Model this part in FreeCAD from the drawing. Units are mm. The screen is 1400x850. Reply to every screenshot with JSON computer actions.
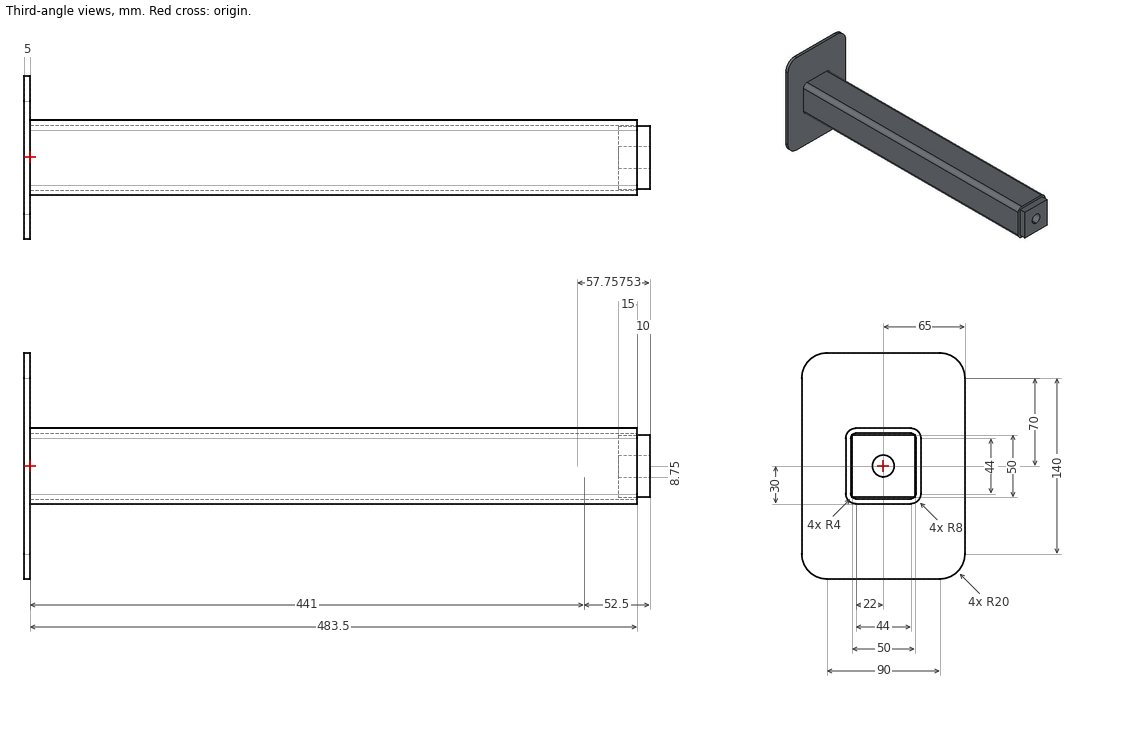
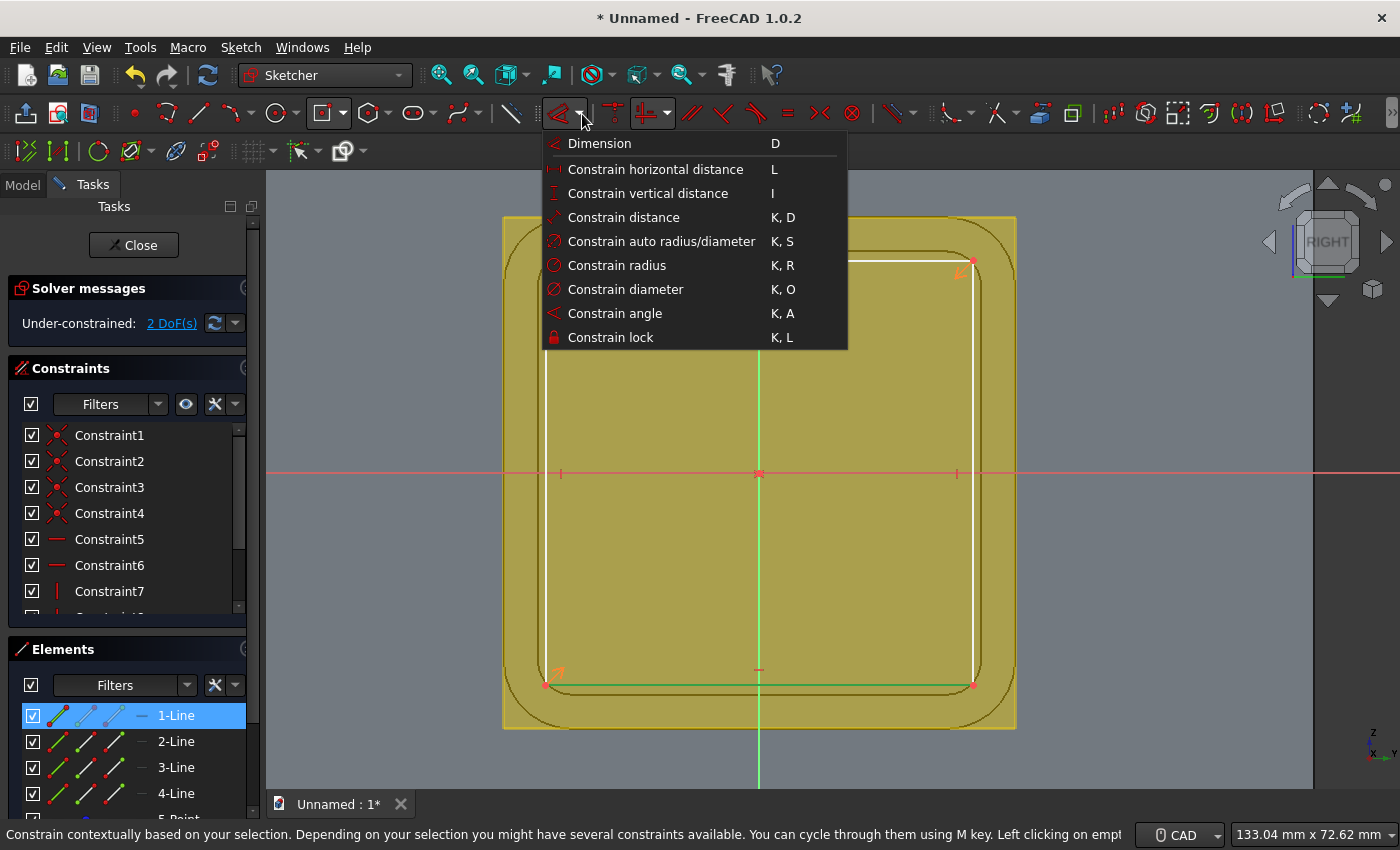
{"action": "left_click", "coordinate": [695, 169]}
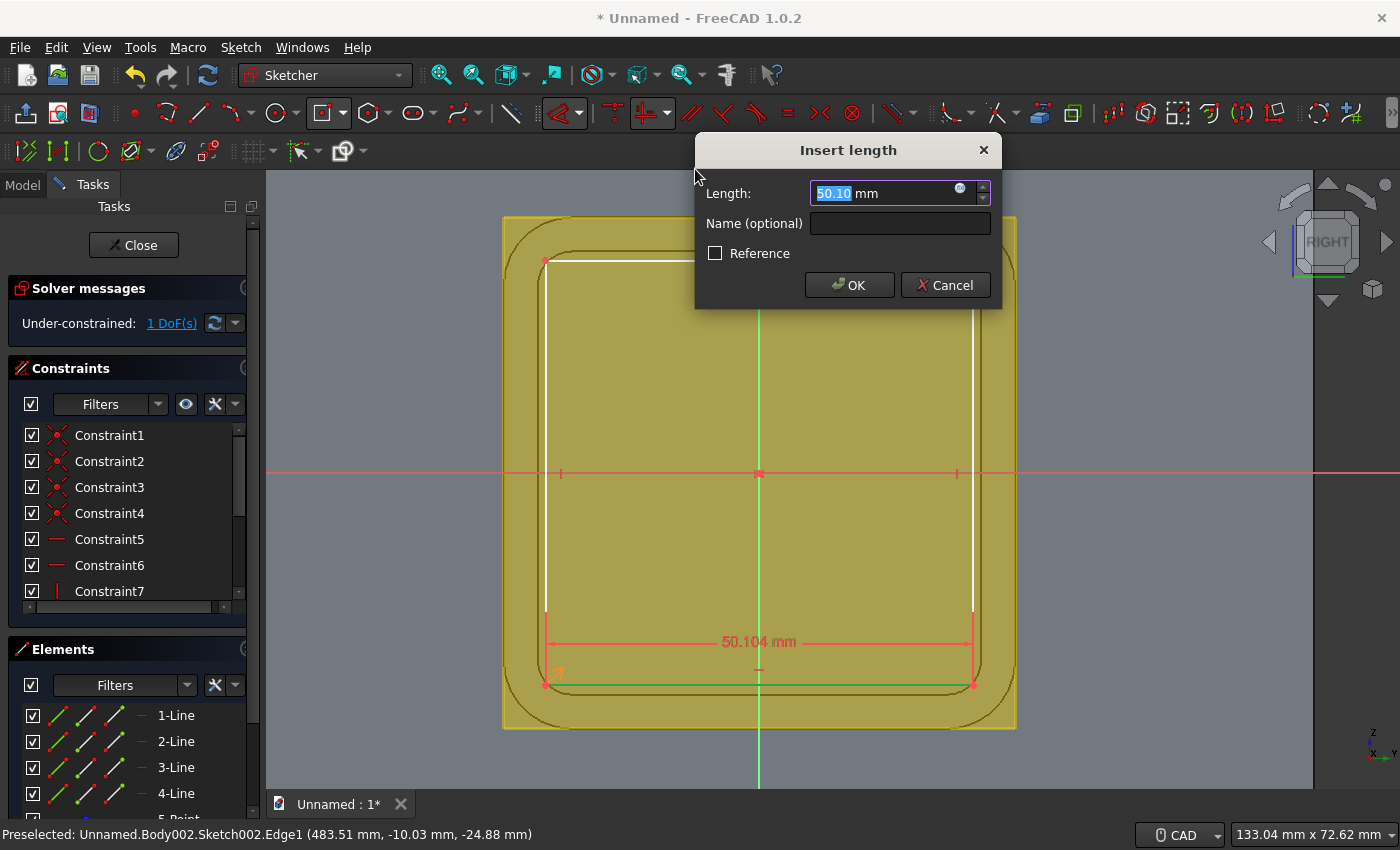
{"action": "type", "text": "50"}
{"action": "key", "text": "Return"}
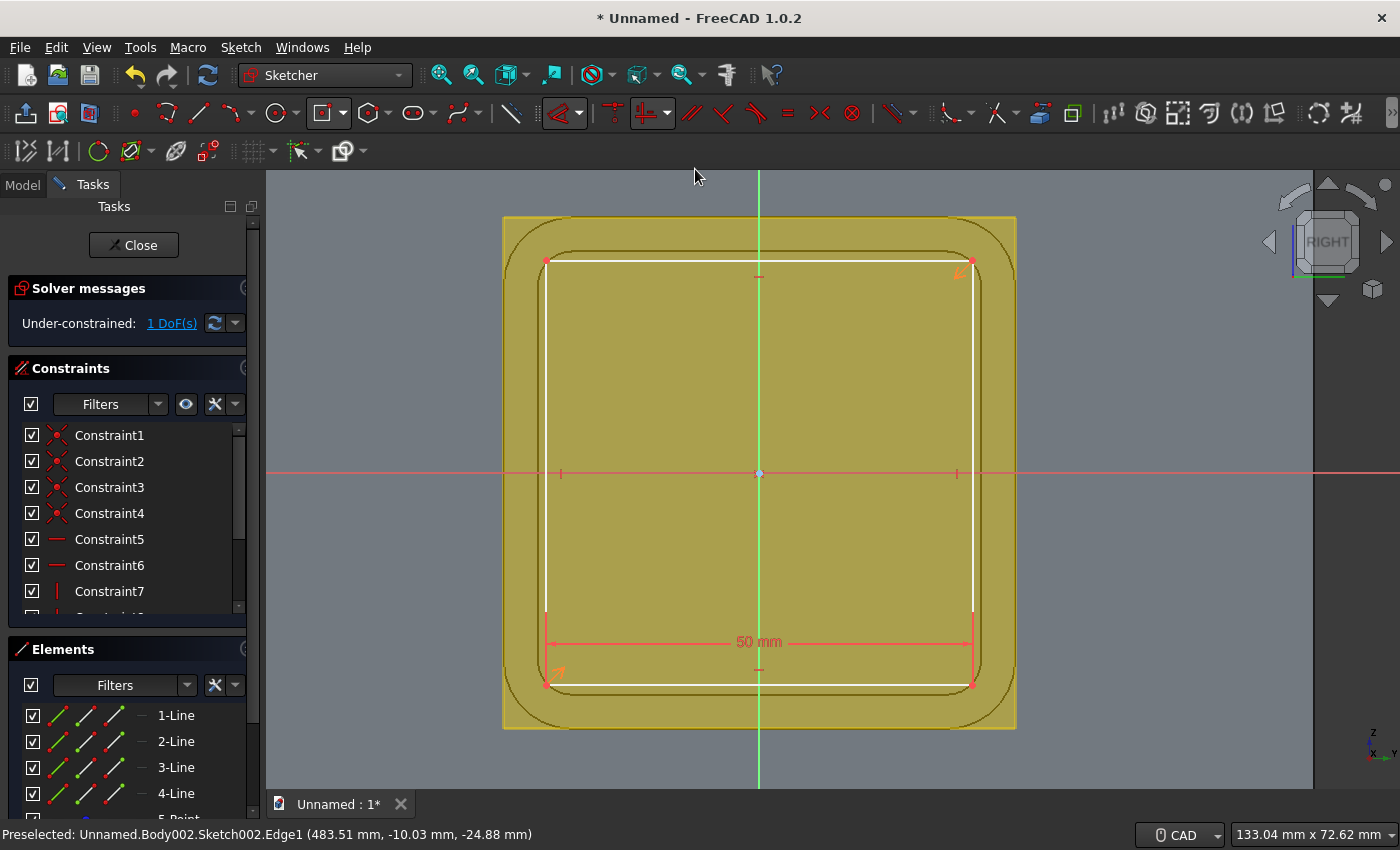
{"action": "left_click", "coordinate": [973, 558]}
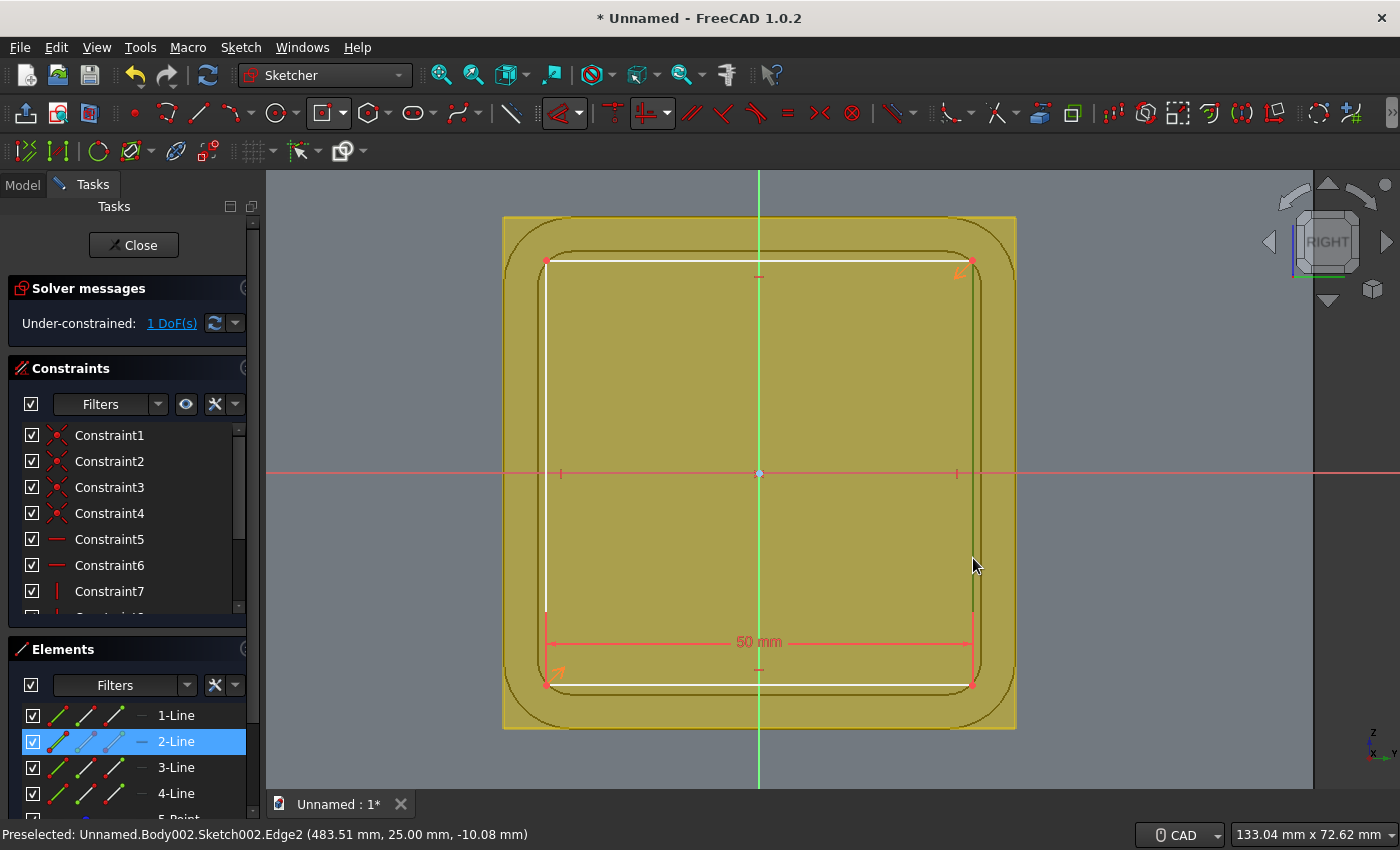
{"action": "key", "text": "i"}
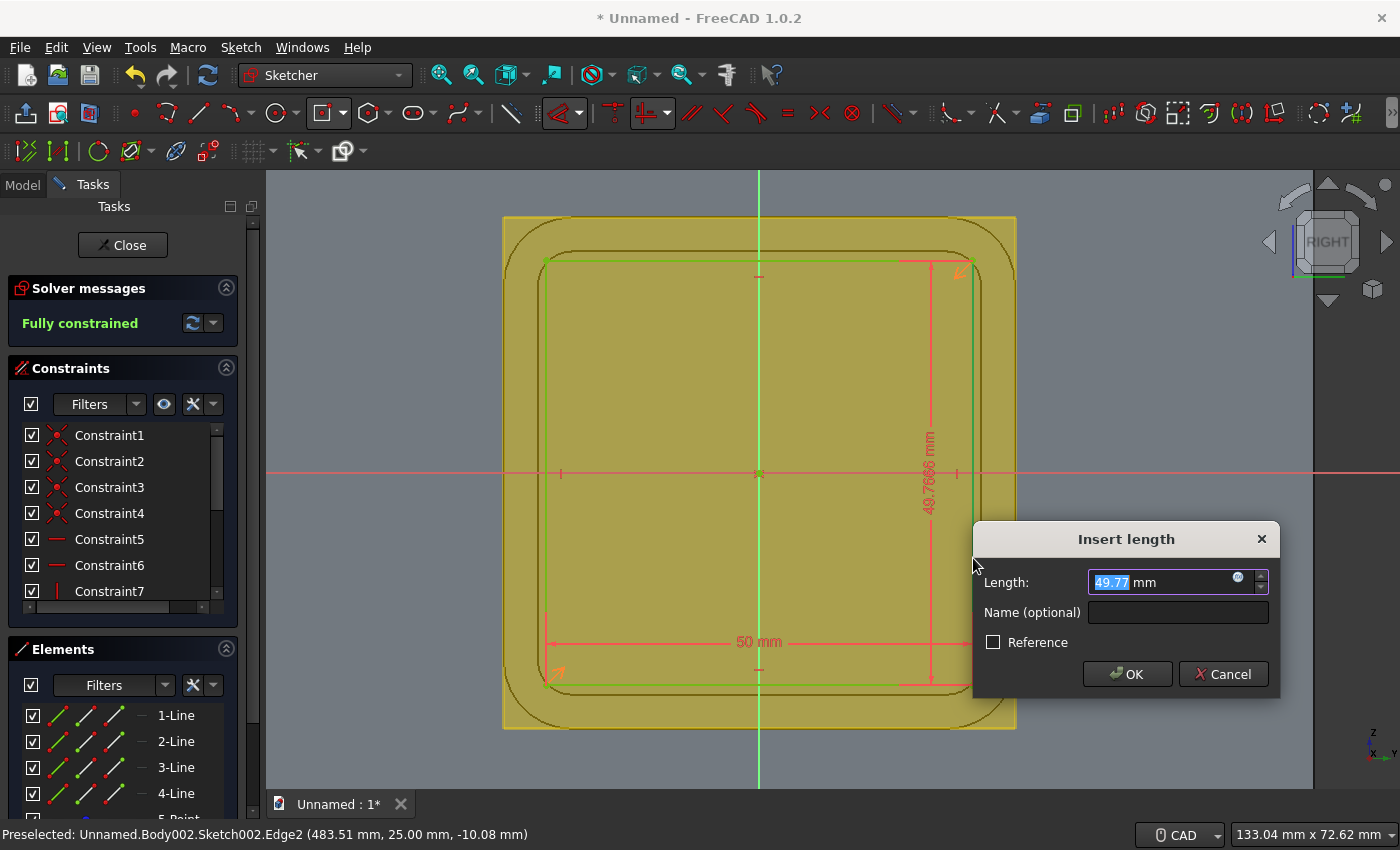
{"action": "type", "text": "50"}
{"action": "key", "text": "Return"}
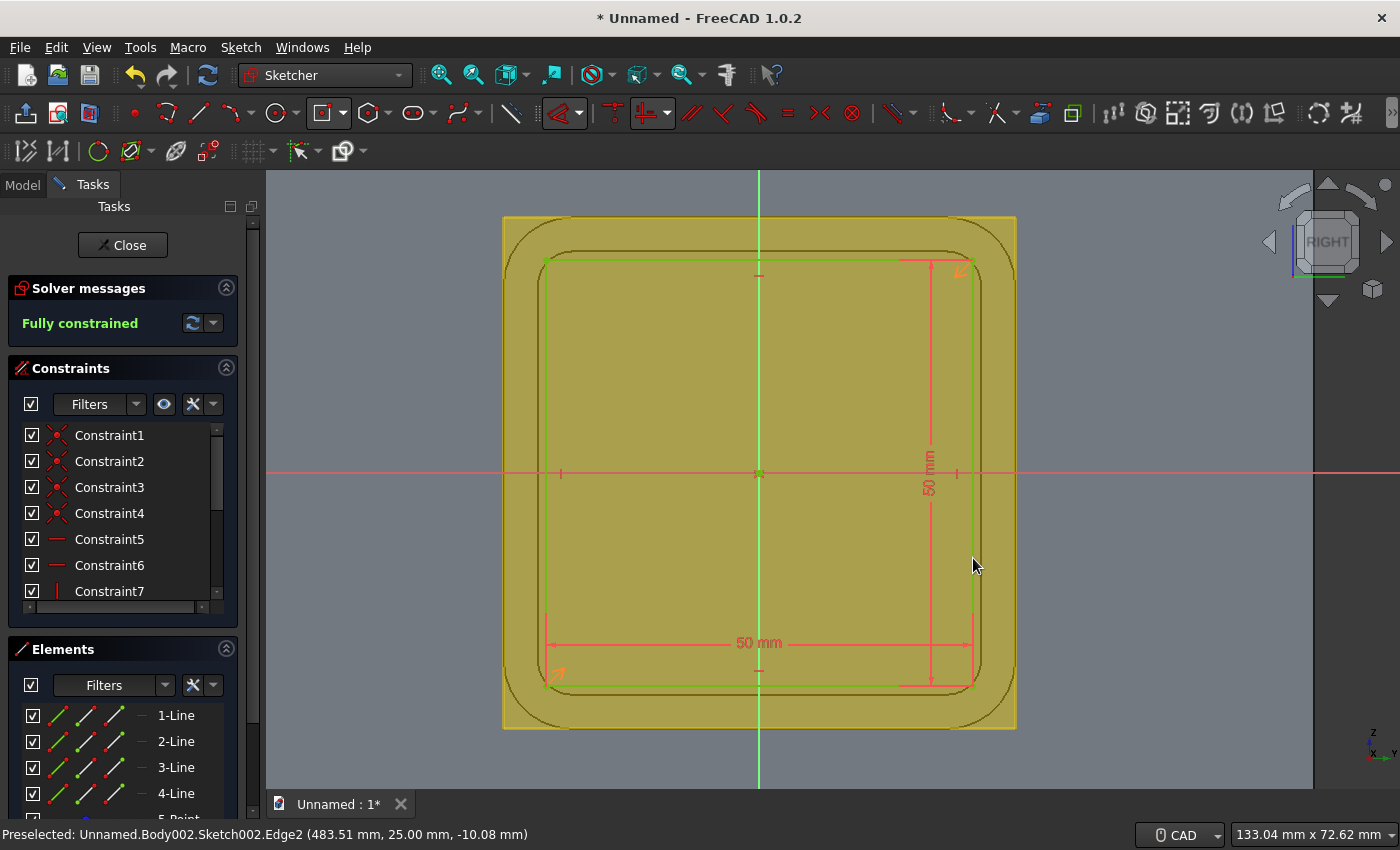
{"action": "left_click", "coordinate": [123, 245]}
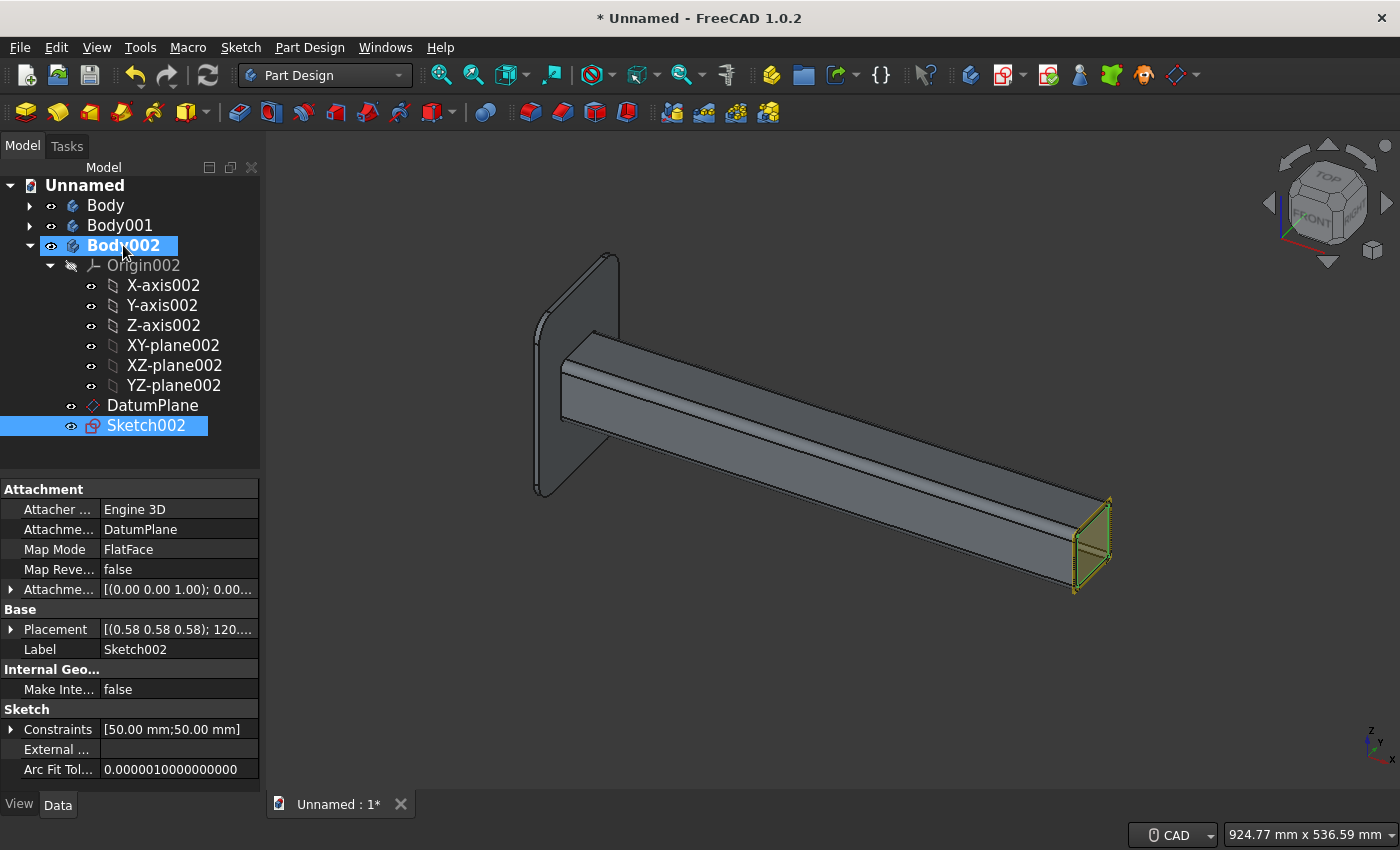
{"action": "left_click", "coordinate": [26, 112]}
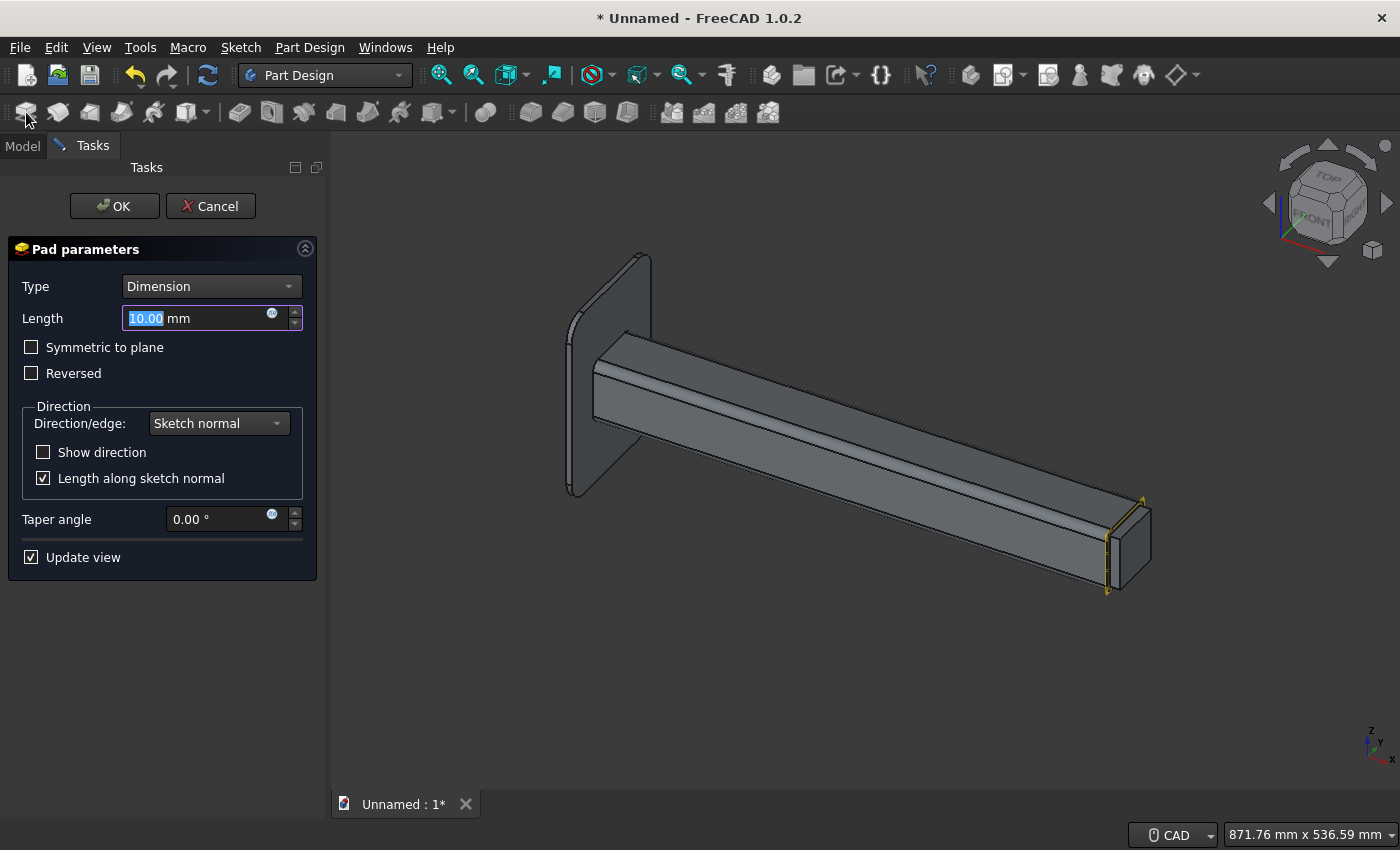
{"action": "left_click", "coordinate": [212, 286]}